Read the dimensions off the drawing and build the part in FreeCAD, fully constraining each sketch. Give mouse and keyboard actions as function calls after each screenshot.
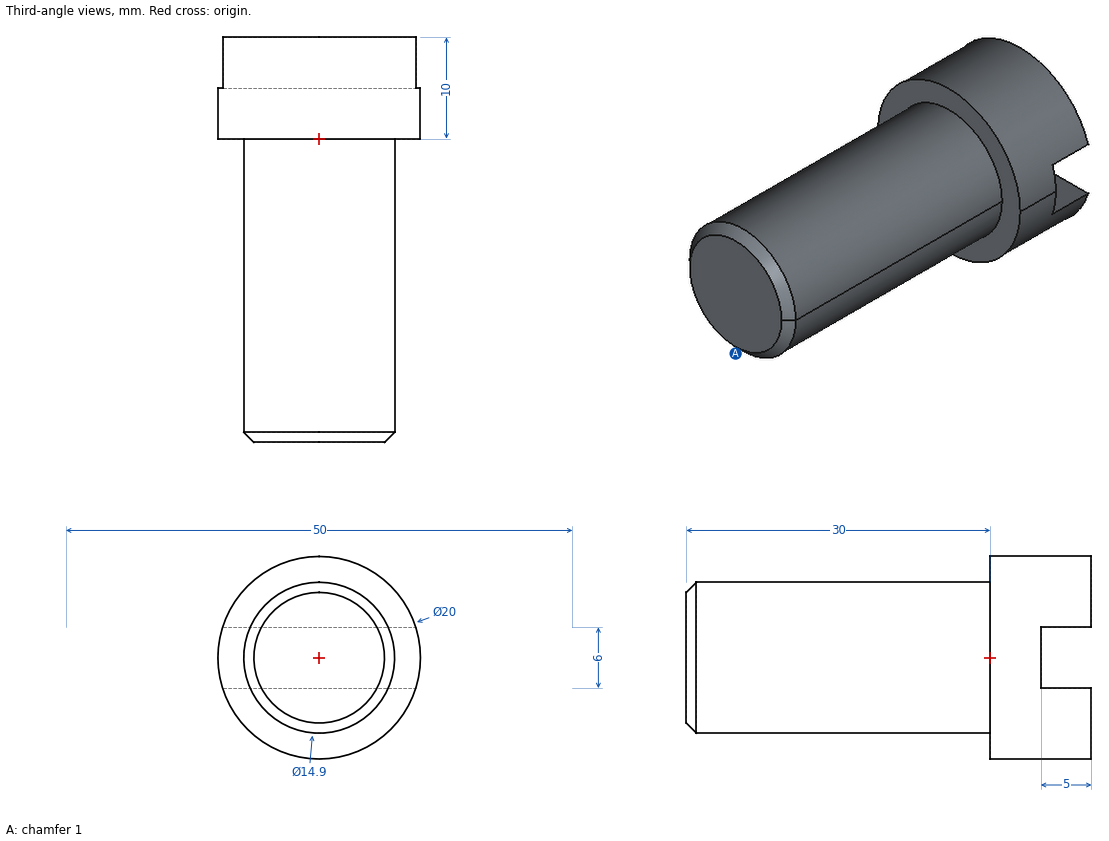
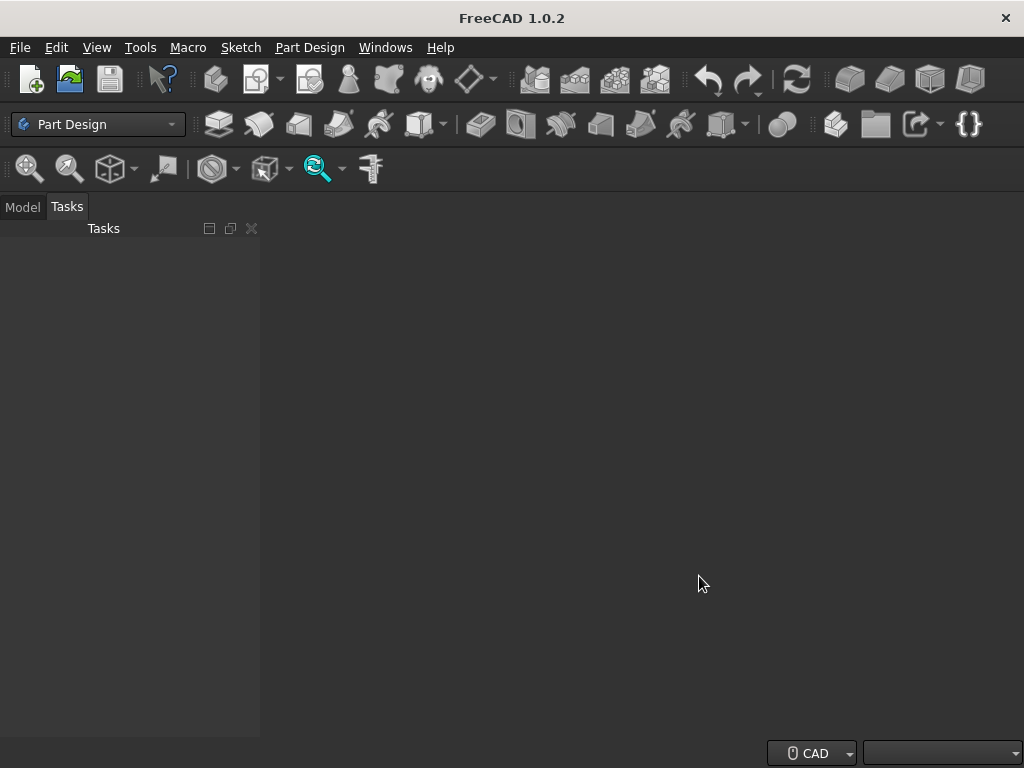
click(30, 80)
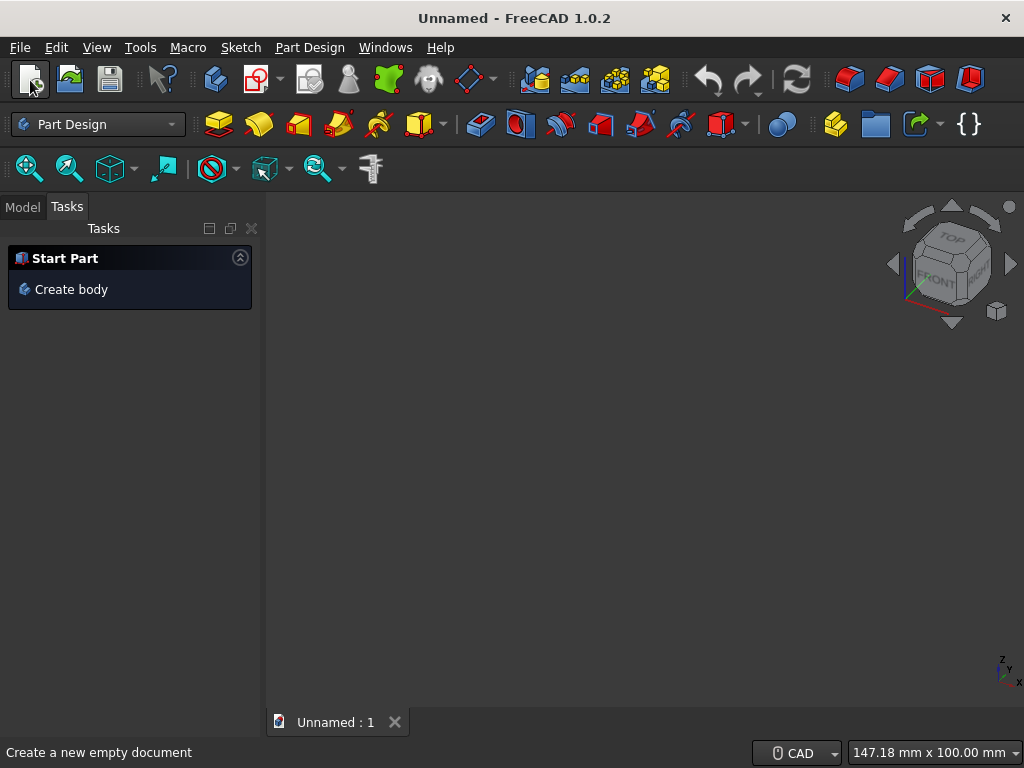
click(256, 80)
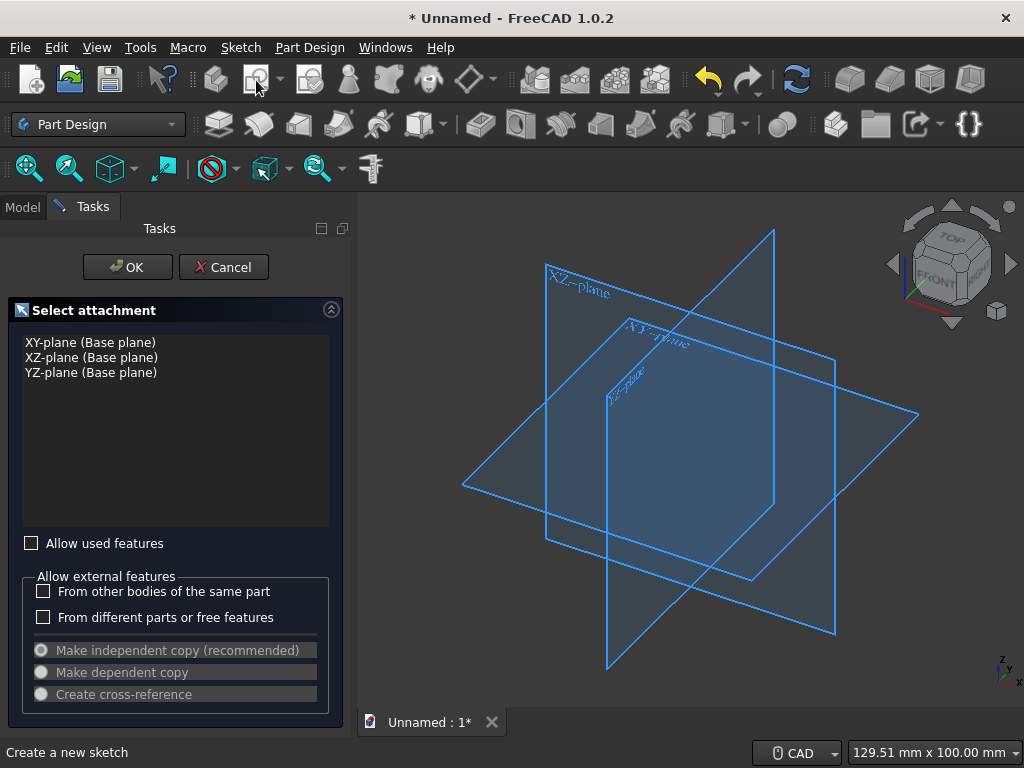
click(82, 358)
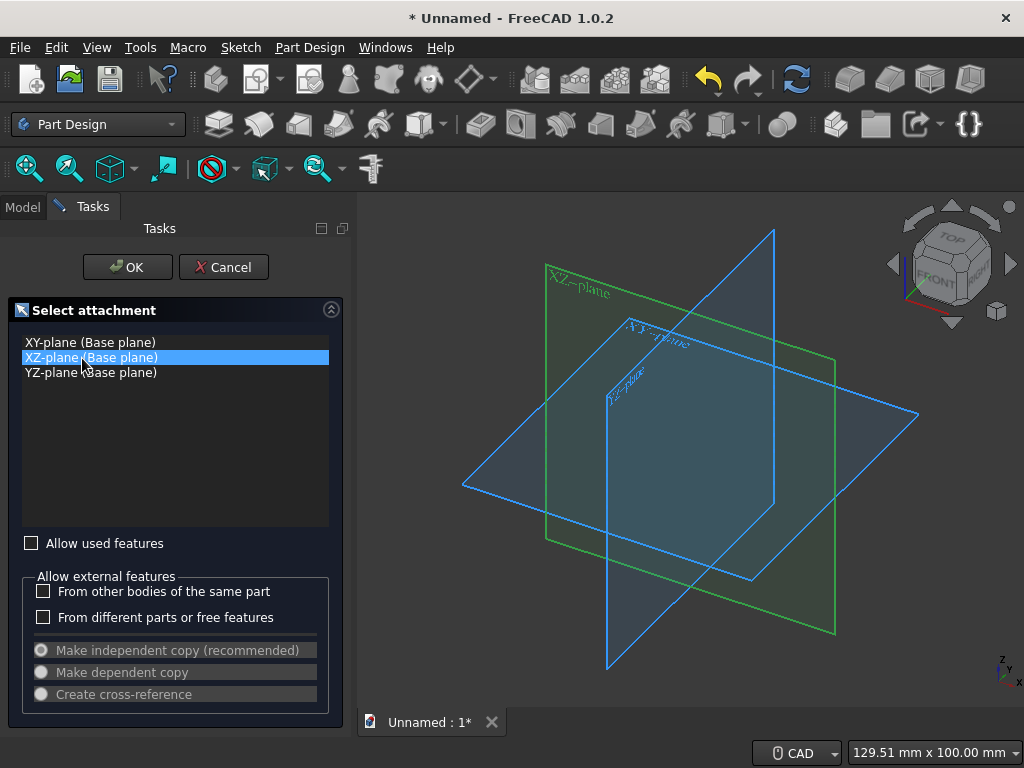
click(128, 267)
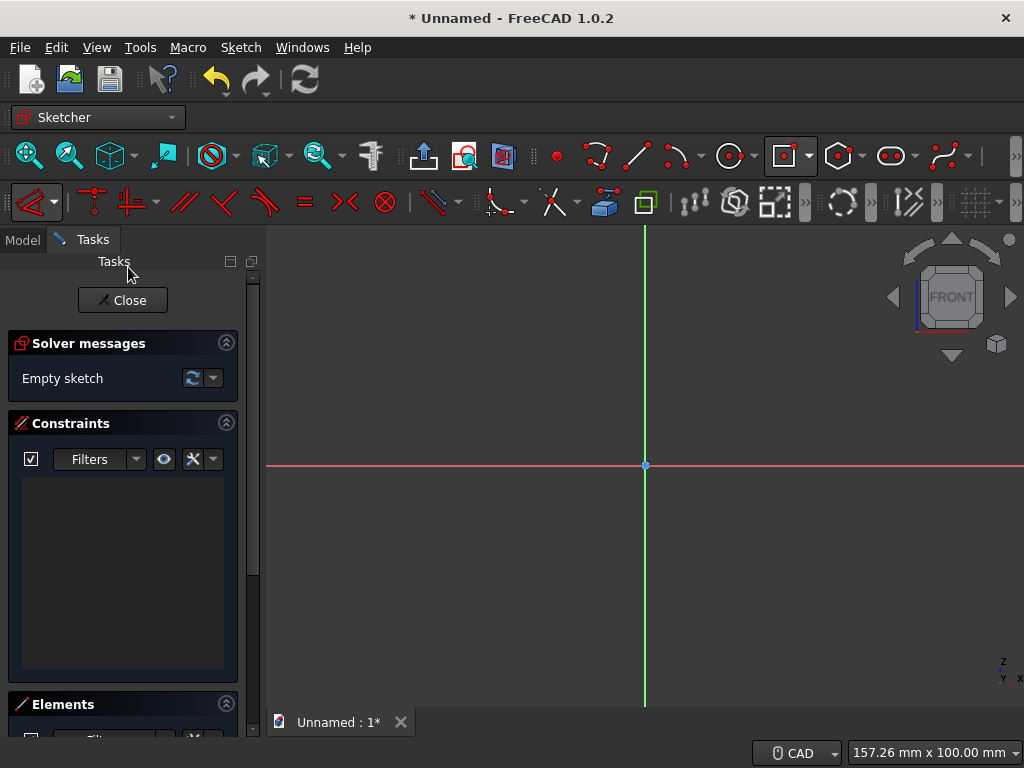
scroll(667, 466, up, 7)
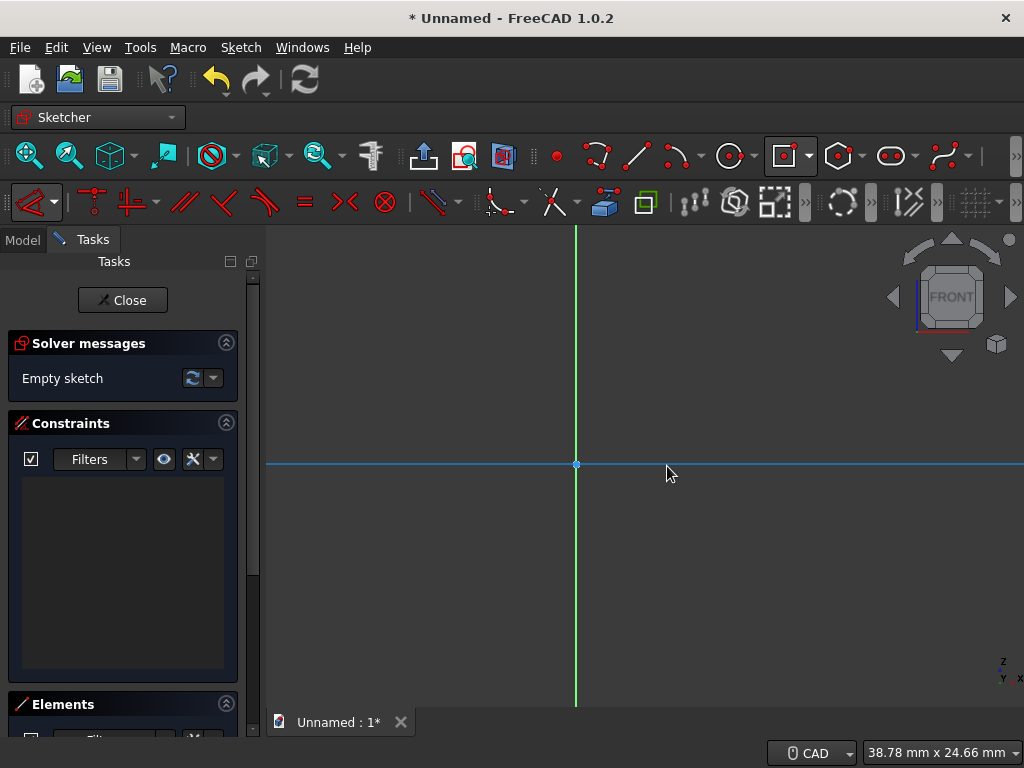
click(730, 156)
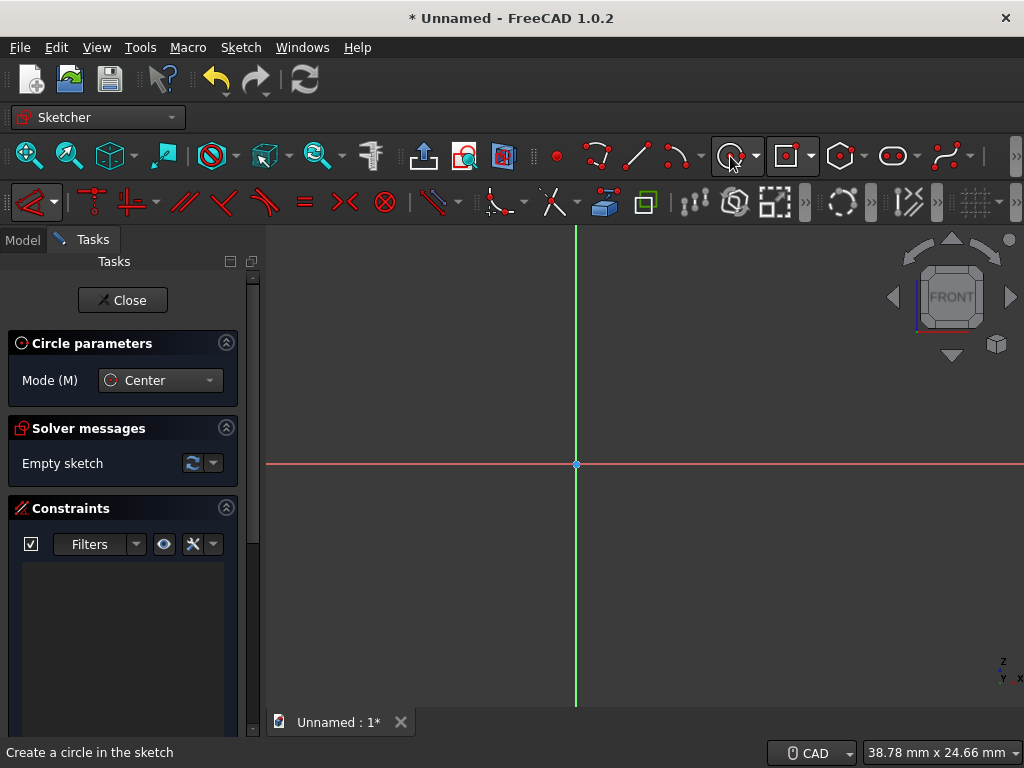
click(576, 464)
move(679, 362)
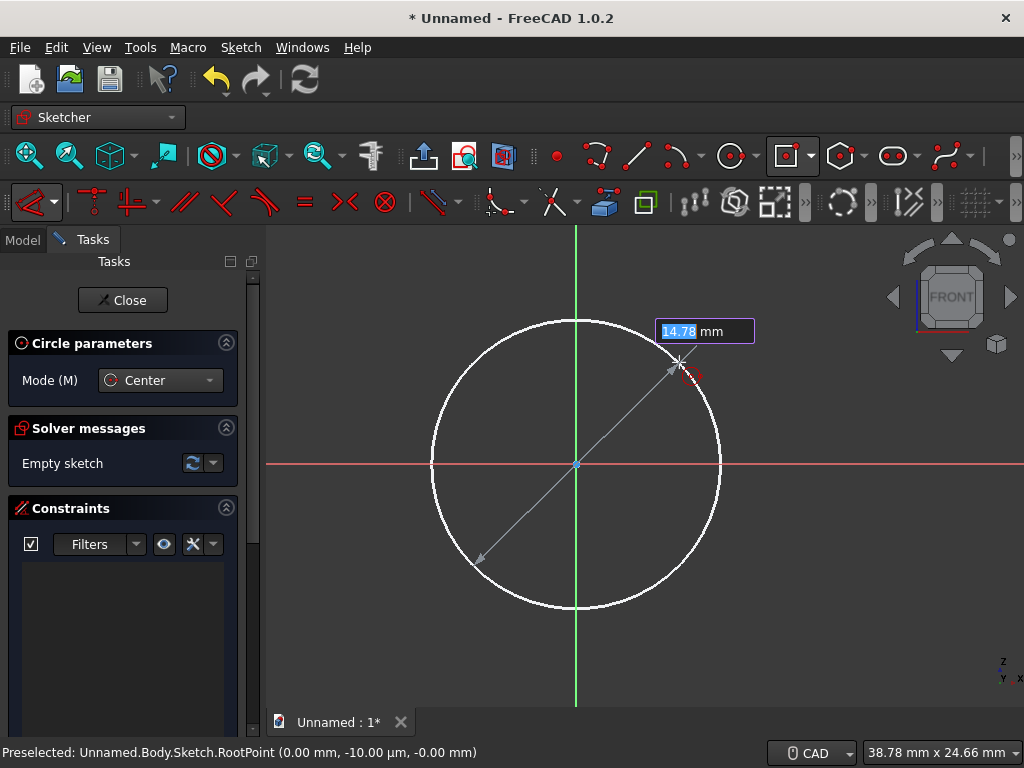
text(14.9)
key(Return)
key(Escape)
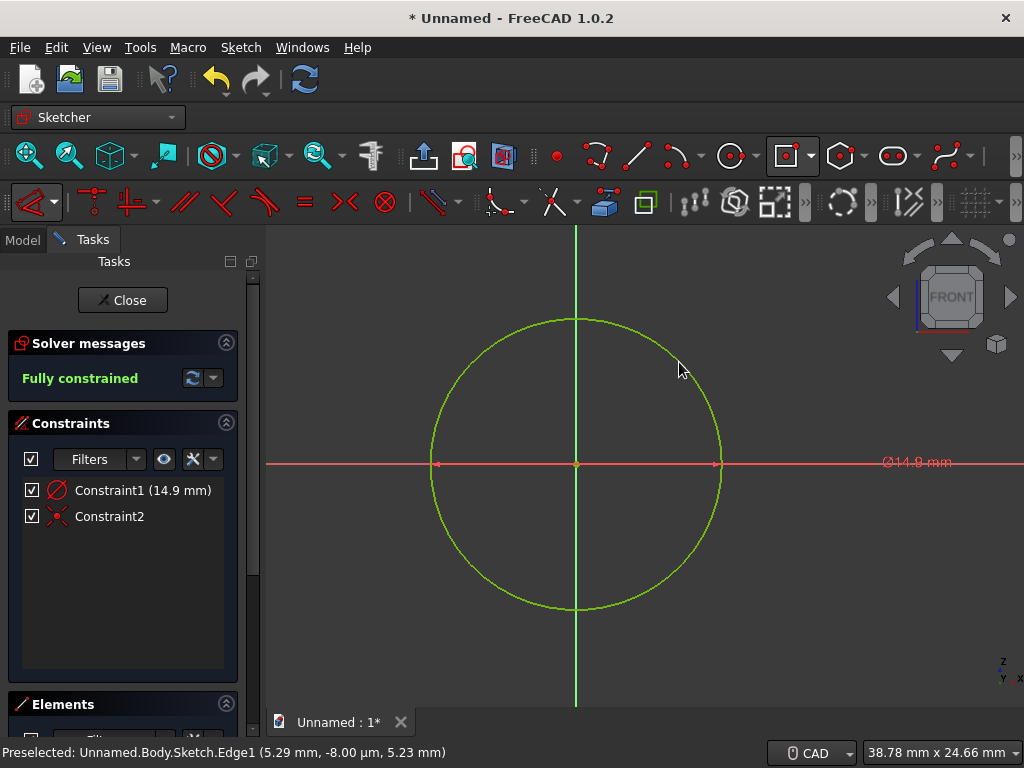
click(123, 300)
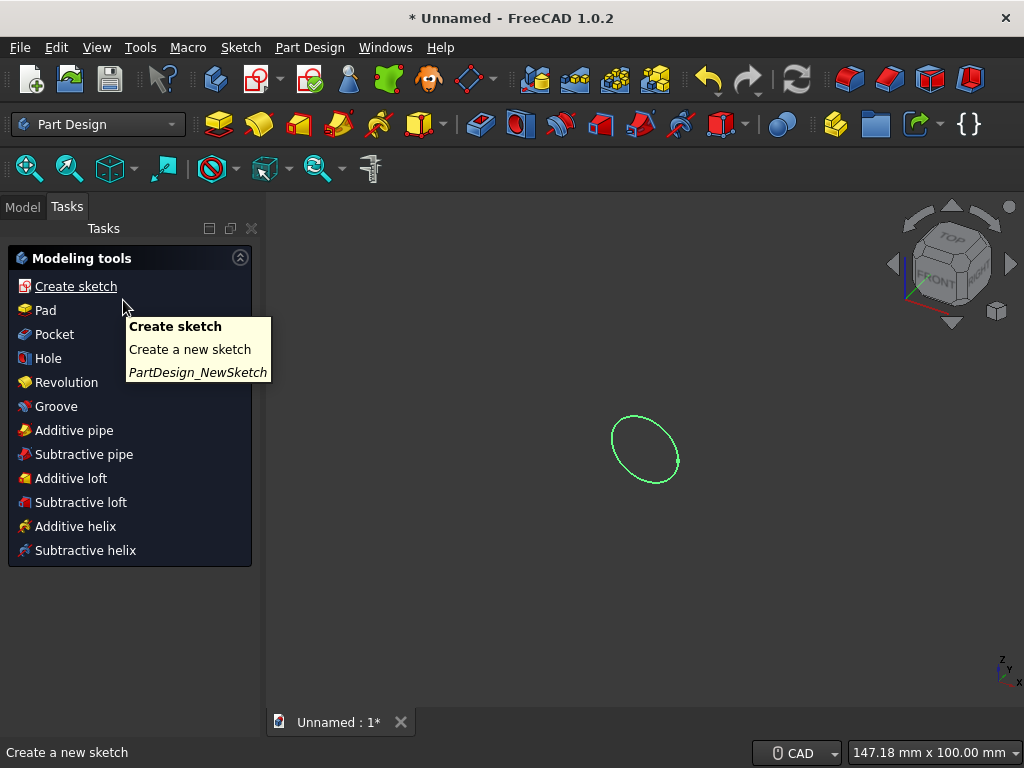
click(220, 124)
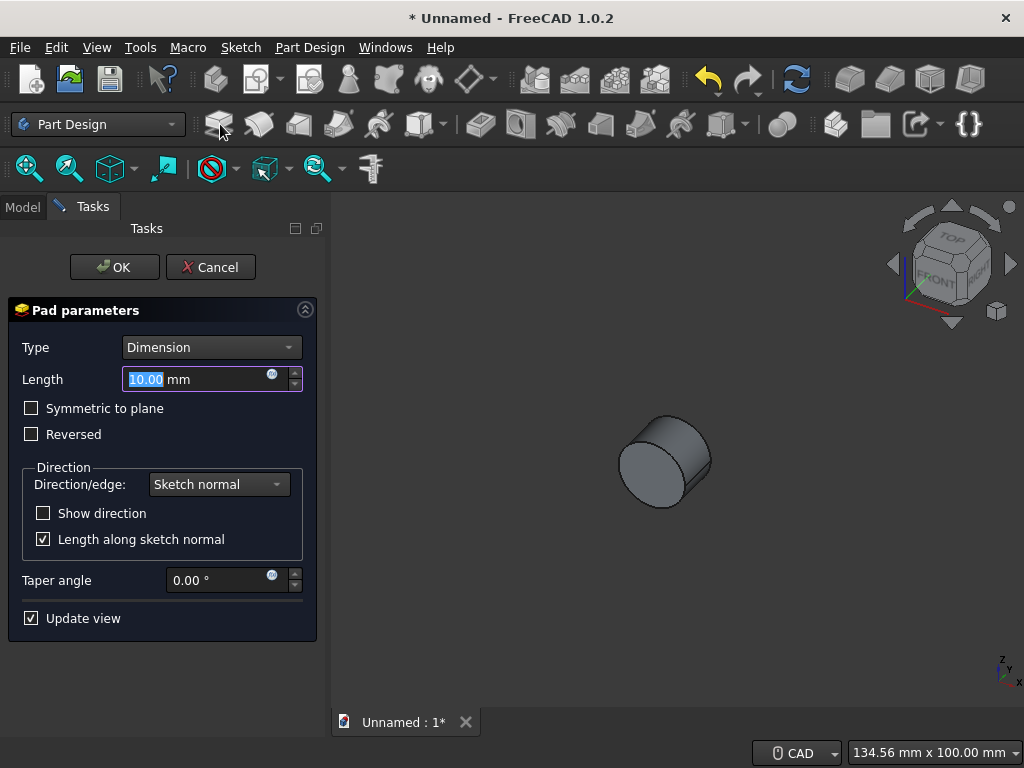
text(30)
key(Tab)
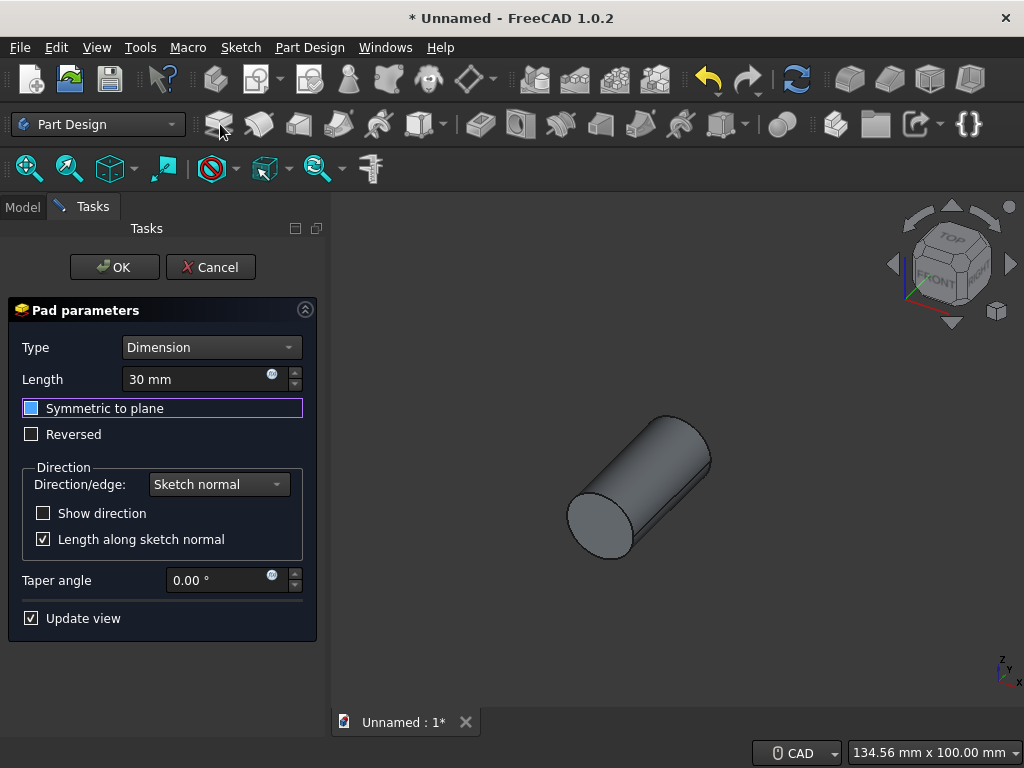
click(115, 267)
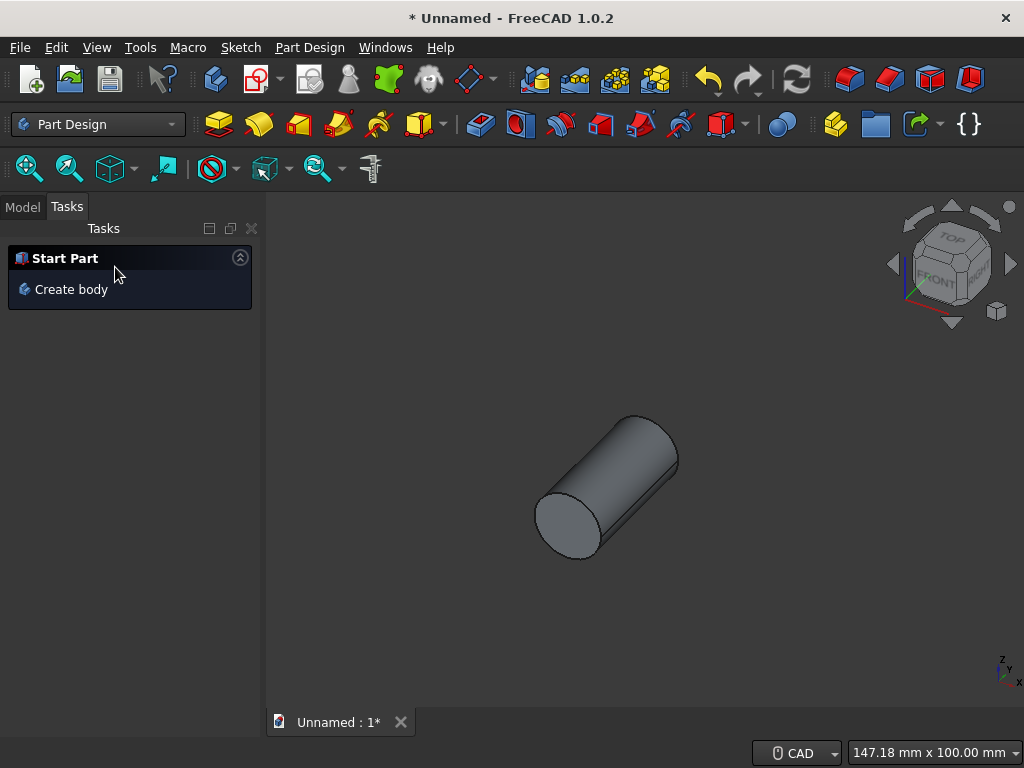
click(30, 170)